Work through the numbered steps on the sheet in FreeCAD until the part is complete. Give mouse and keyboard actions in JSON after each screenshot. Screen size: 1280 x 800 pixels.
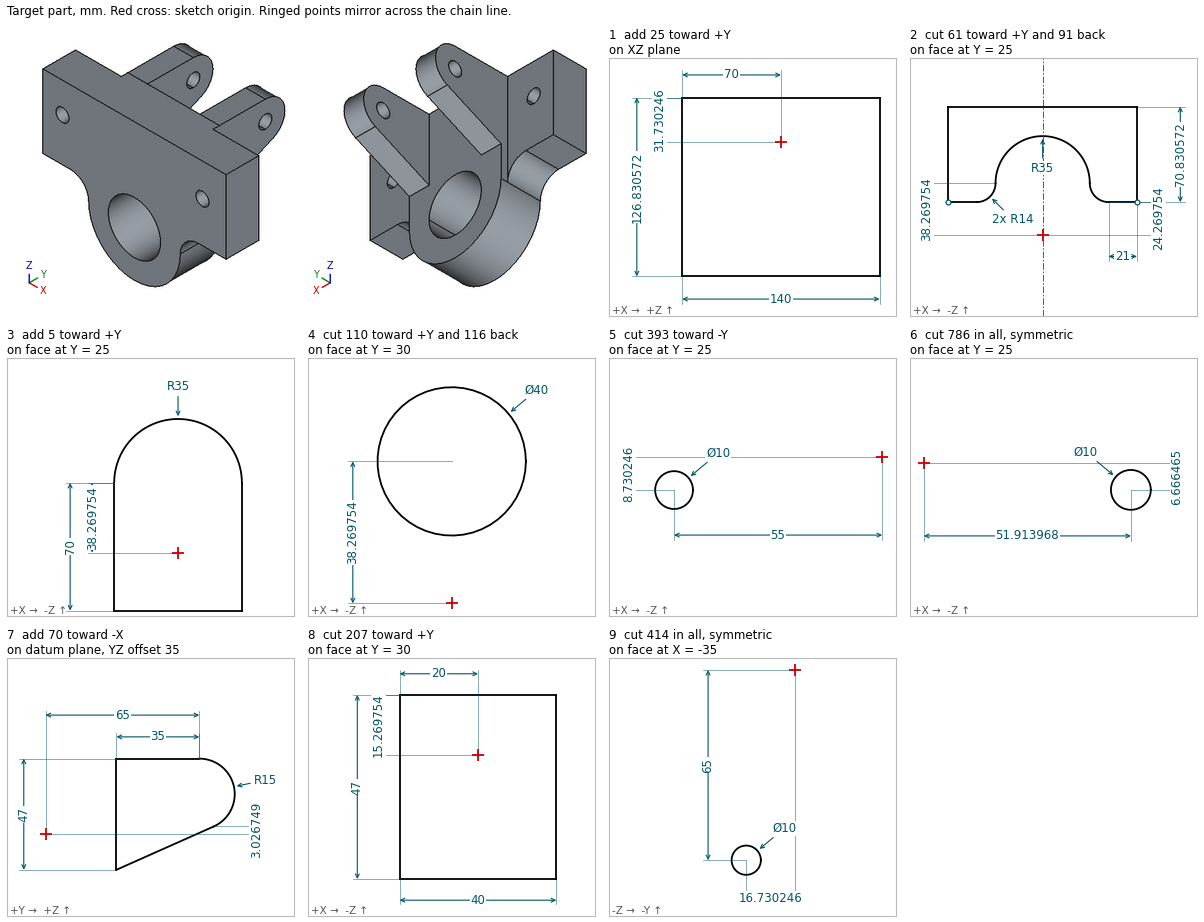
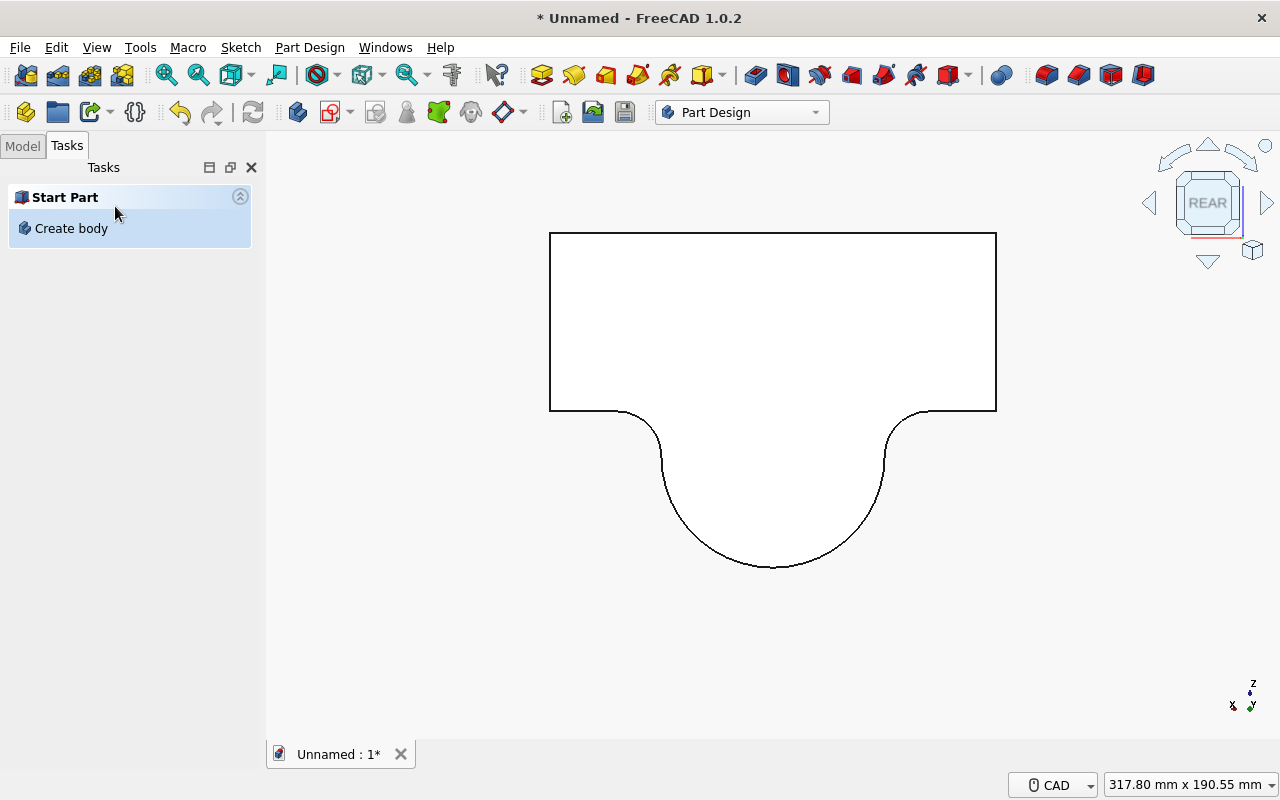
{"action": "left_click", "coordinate": [773, 399]}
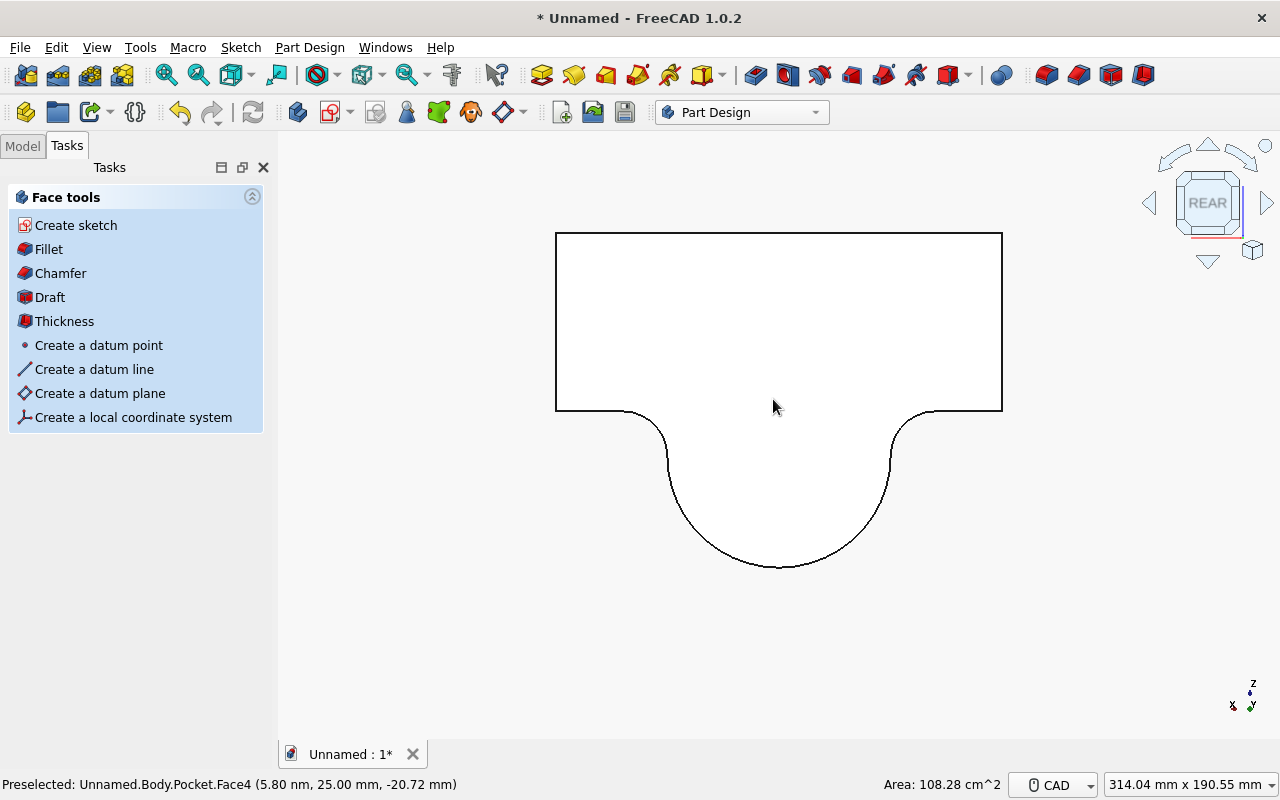
{"action": "left_click", "coordinate": [330, 112]}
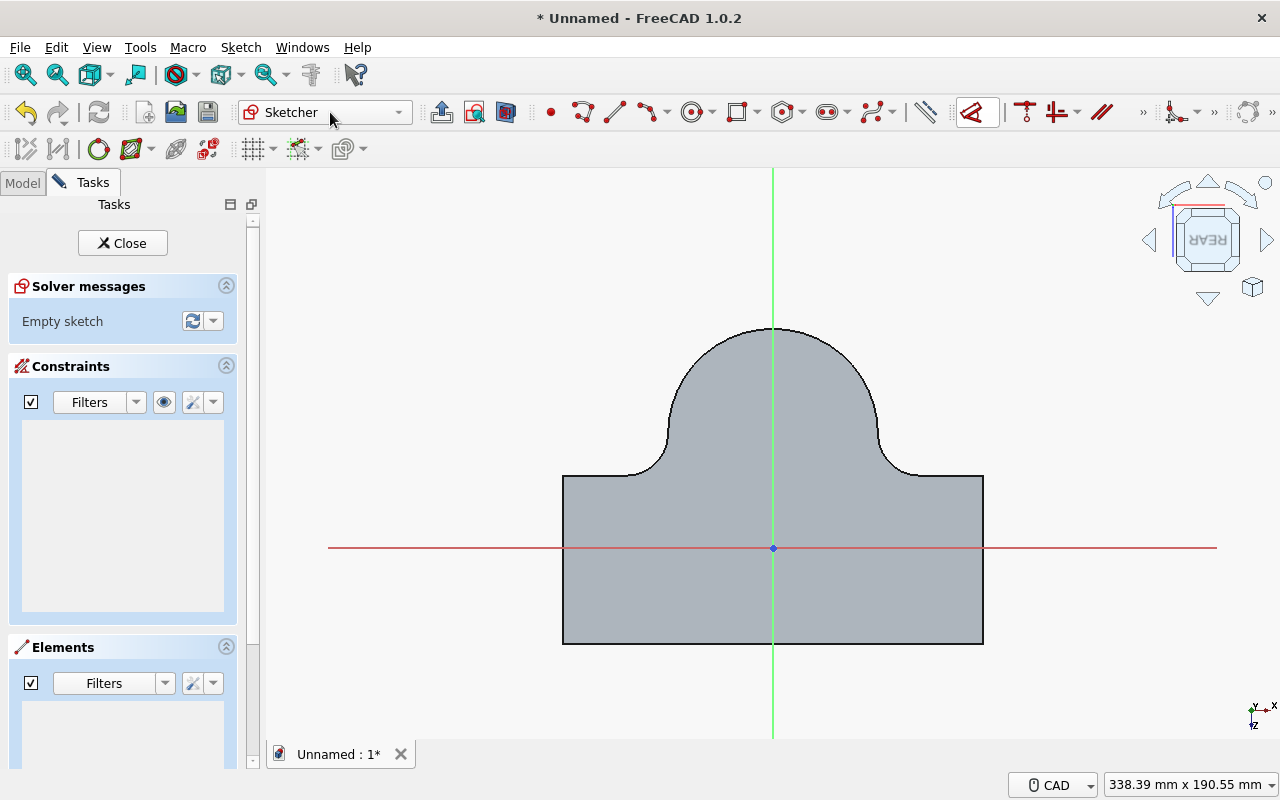
{"action": "left_click", "coordinate": [584, 112]}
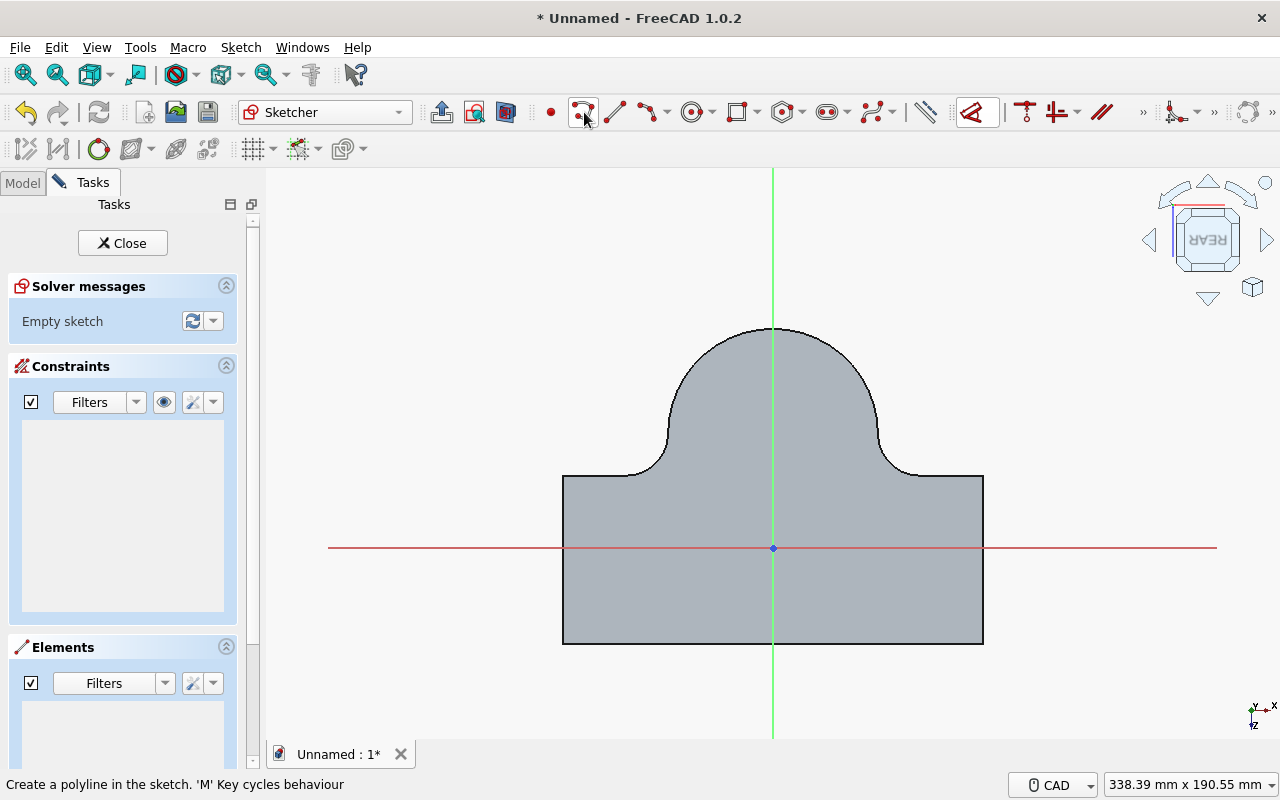
{"action": "left_click", "coordinate": [668, 434]}
{"action": "left_click", "coordinate": [668, 644]}
{"action": "left_click", "coordinate": [878, 644]}
{"action": "left_click", "coordinate": [878, 434]}
{"action": "right_click", "coordinate": [878, 434]}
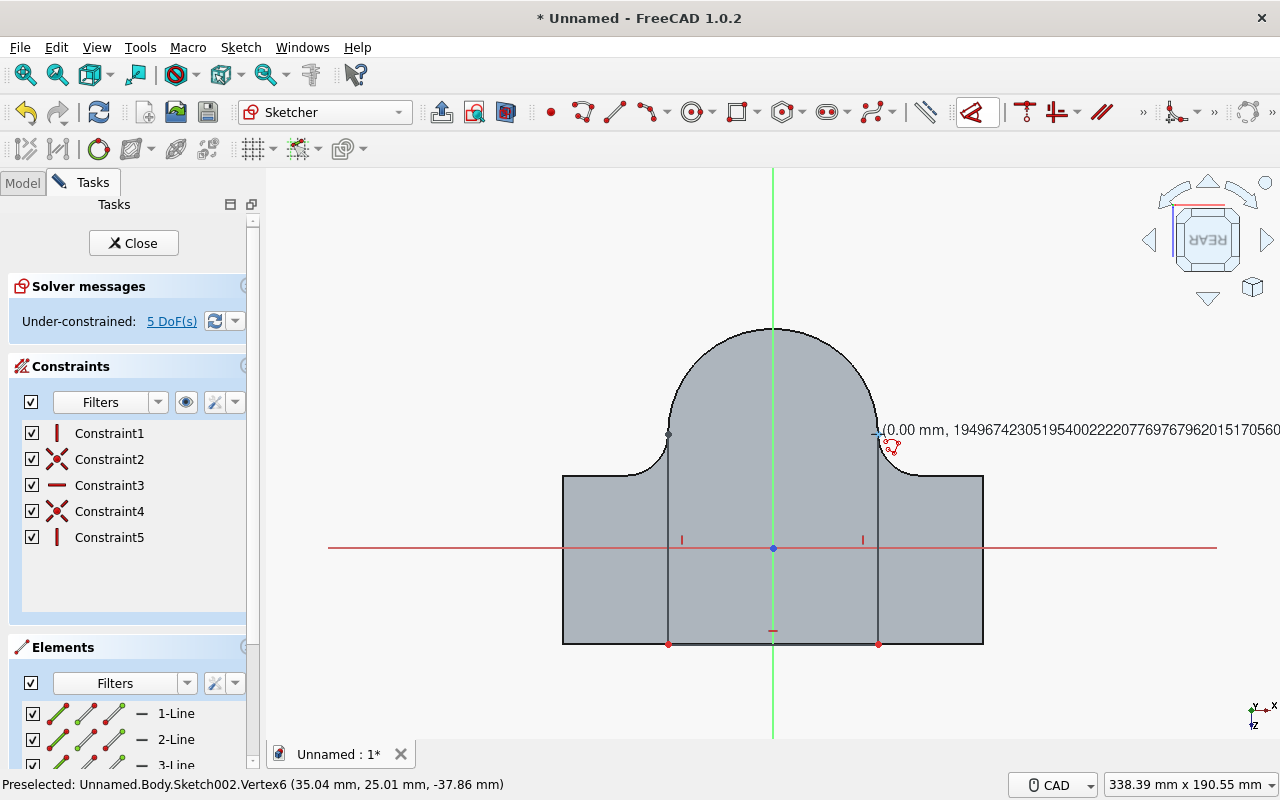
{"action": "left_click", "coordinate": [648, 112]}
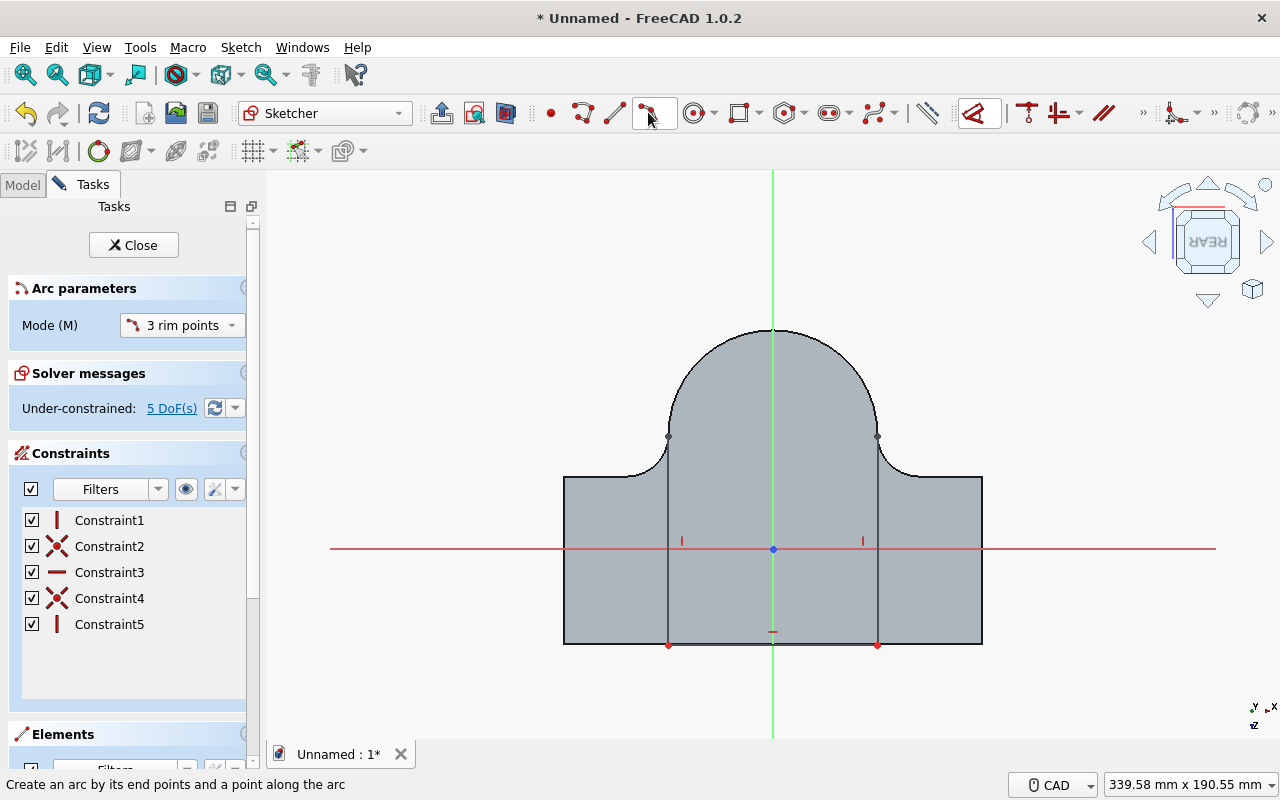
{"action": "left_click", "coordinate": [878, 436]}
{"action": "left_click", "coordinate": [668, 436]}
{"action": "left_click", "coordinate": [805, 335]}
{"action": "key", "text": "Escape"}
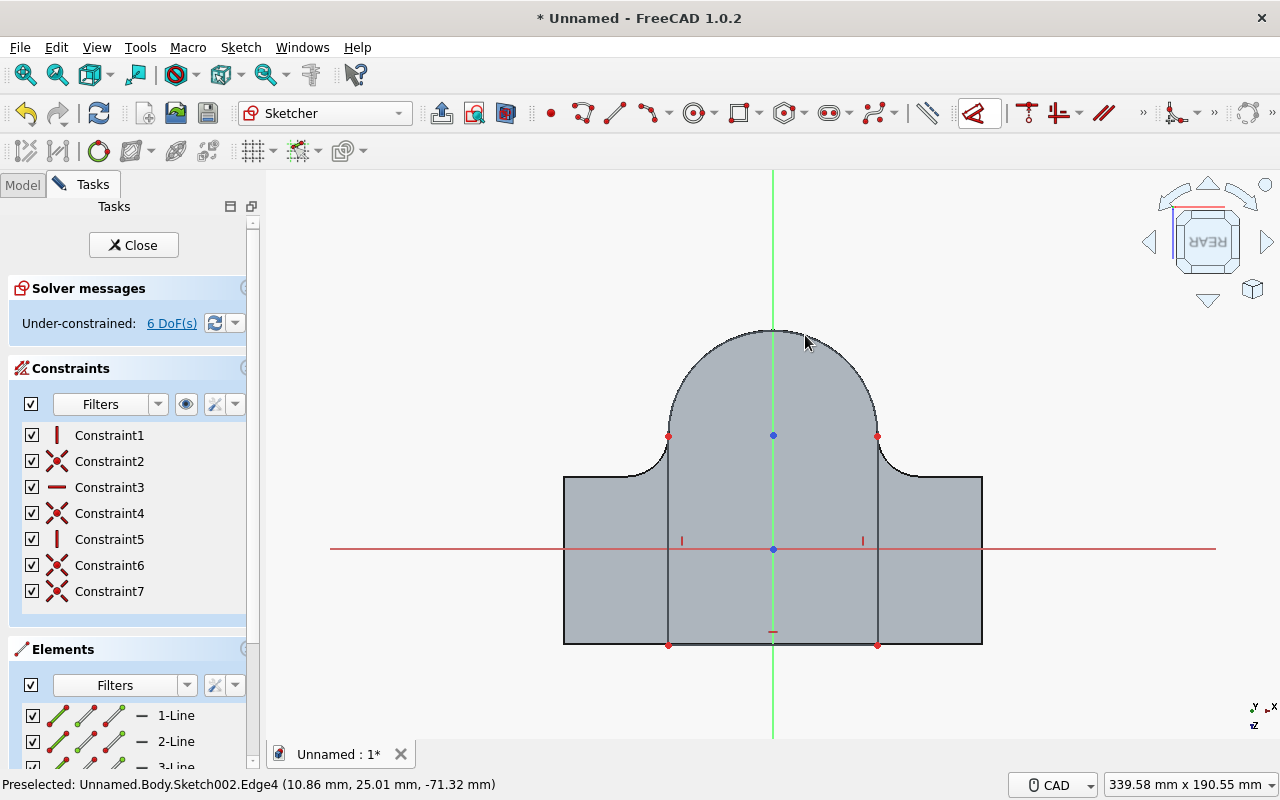
{"action": "left_click", "coordinate": [668, 499]}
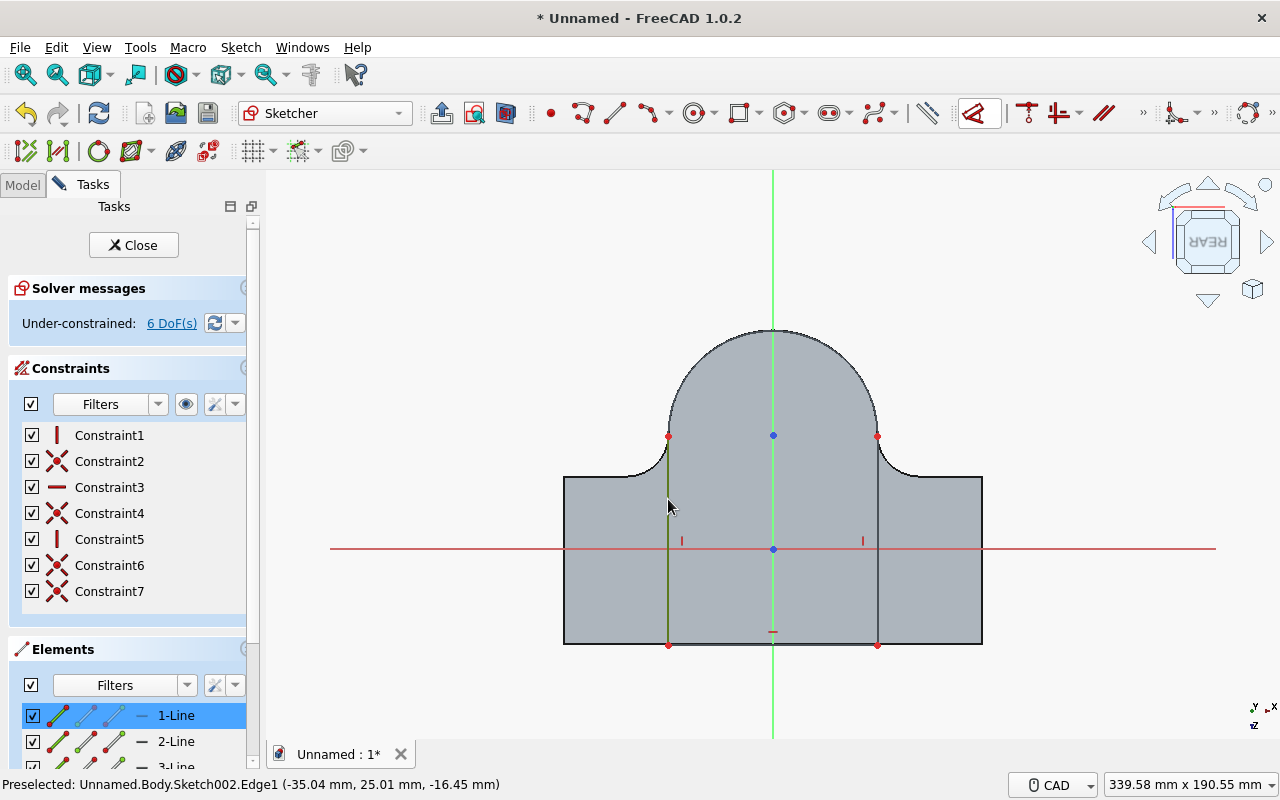
{"action": "left_click", "coordinate": [835, 351]}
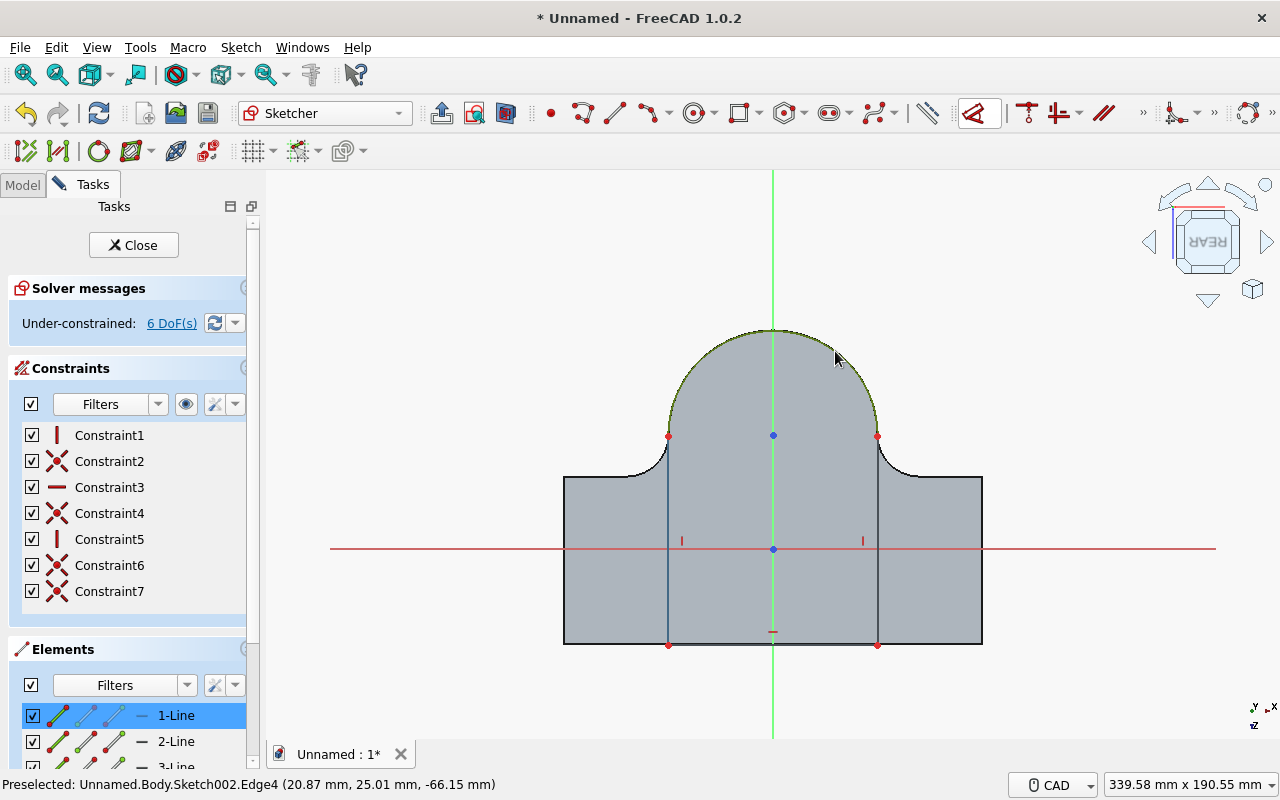
{"action": "key", "text": "t"}